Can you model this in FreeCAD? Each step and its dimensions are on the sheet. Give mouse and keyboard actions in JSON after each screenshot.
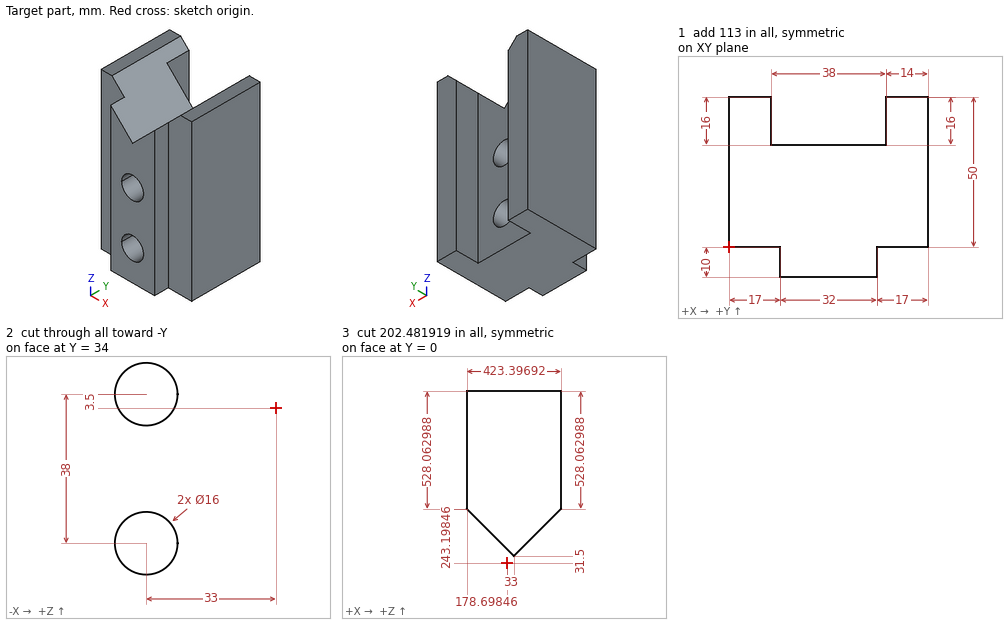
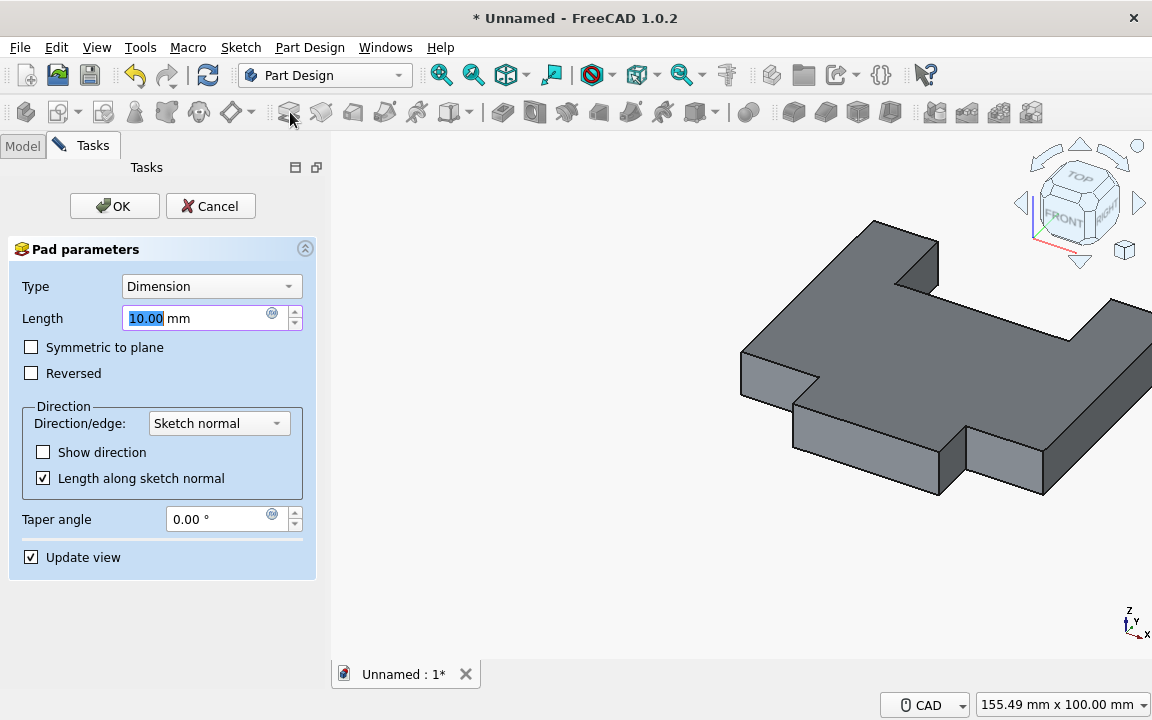
{"action": "type", "text": "113"}
{"action": "key", "text": "Tab"}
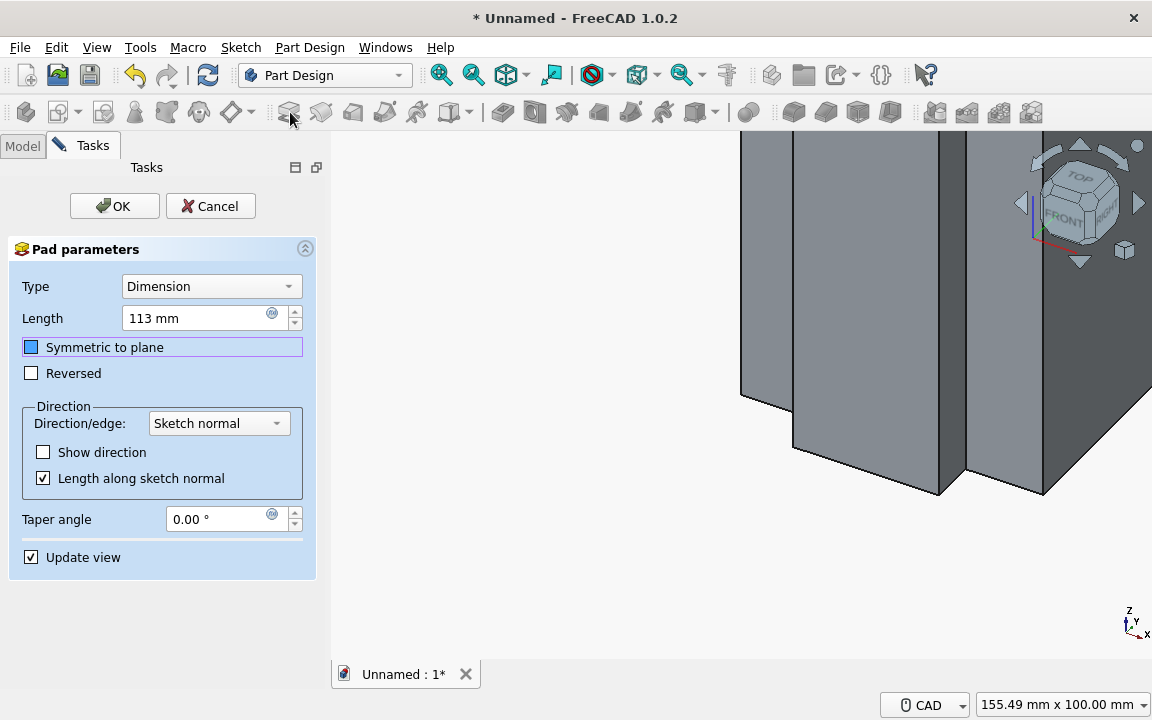
{"action": "left_click", "coordinate": [30, 347]}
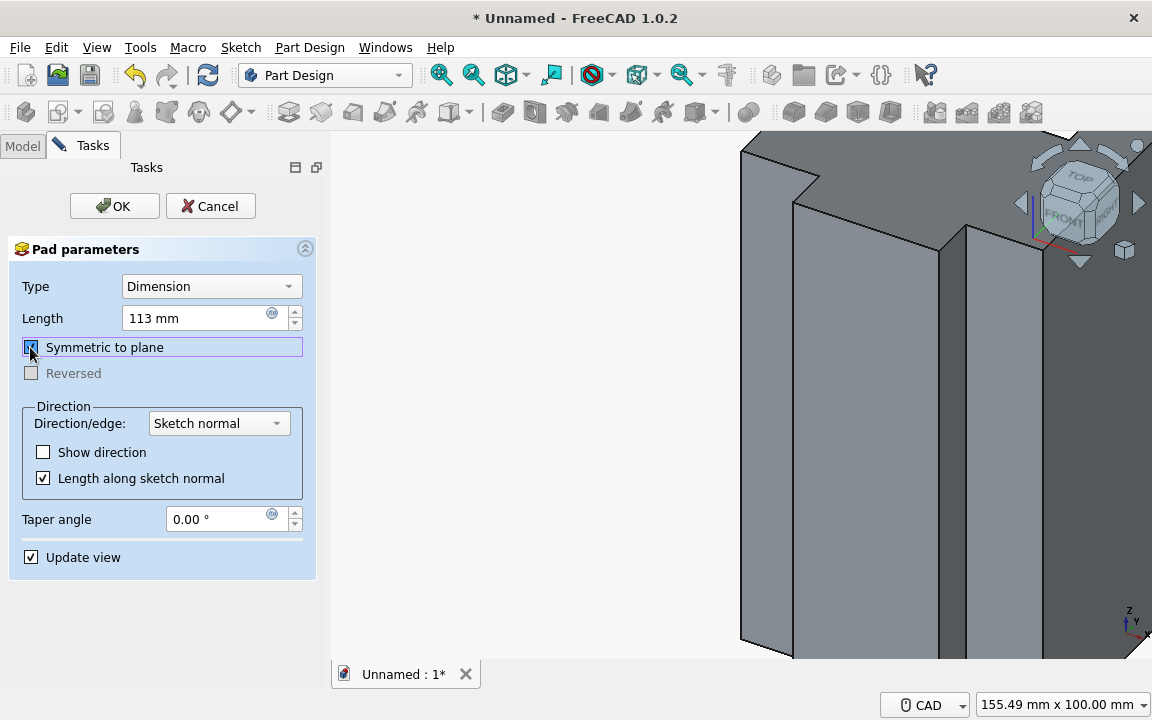
{"action": "left_click", "coordinate": [115, 206]}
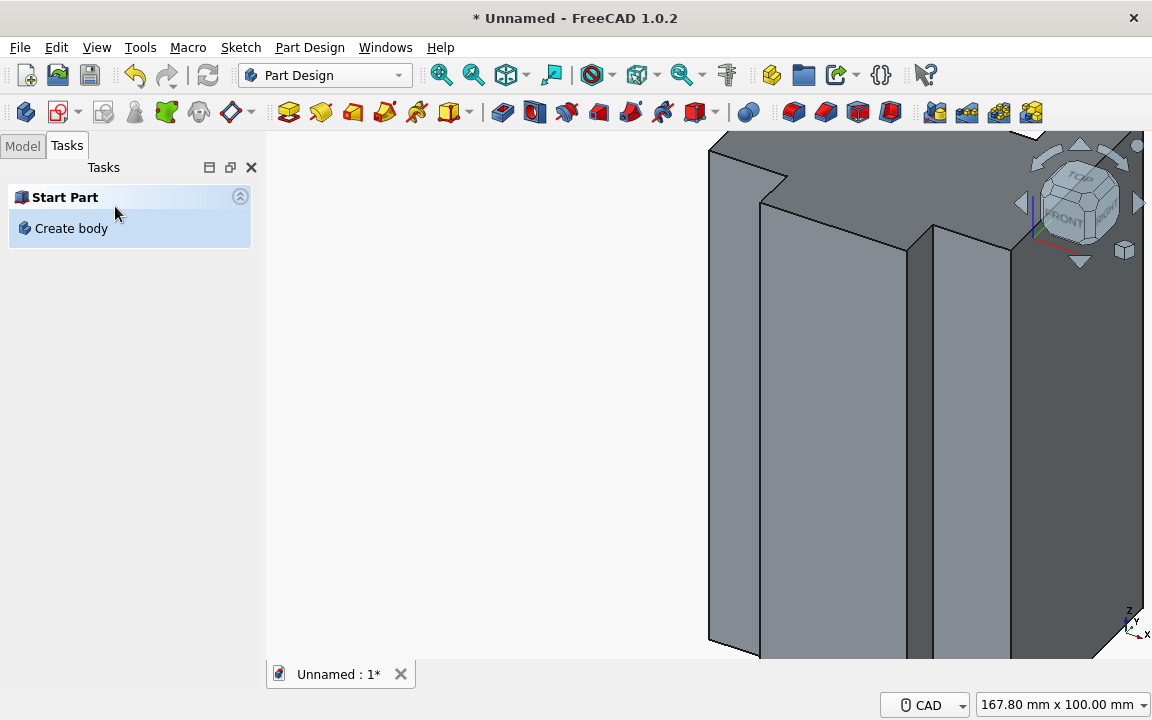
{"action": "left_click", "coordinate": [442, 76]}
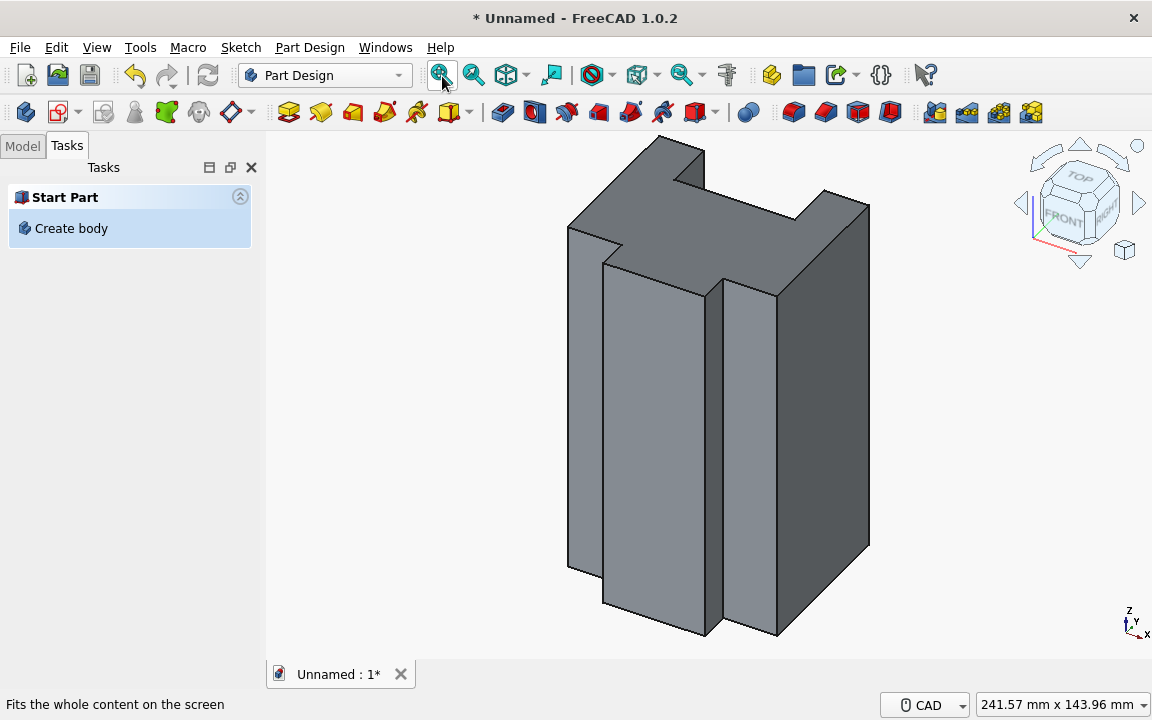
{"action": "key", "text": "4"}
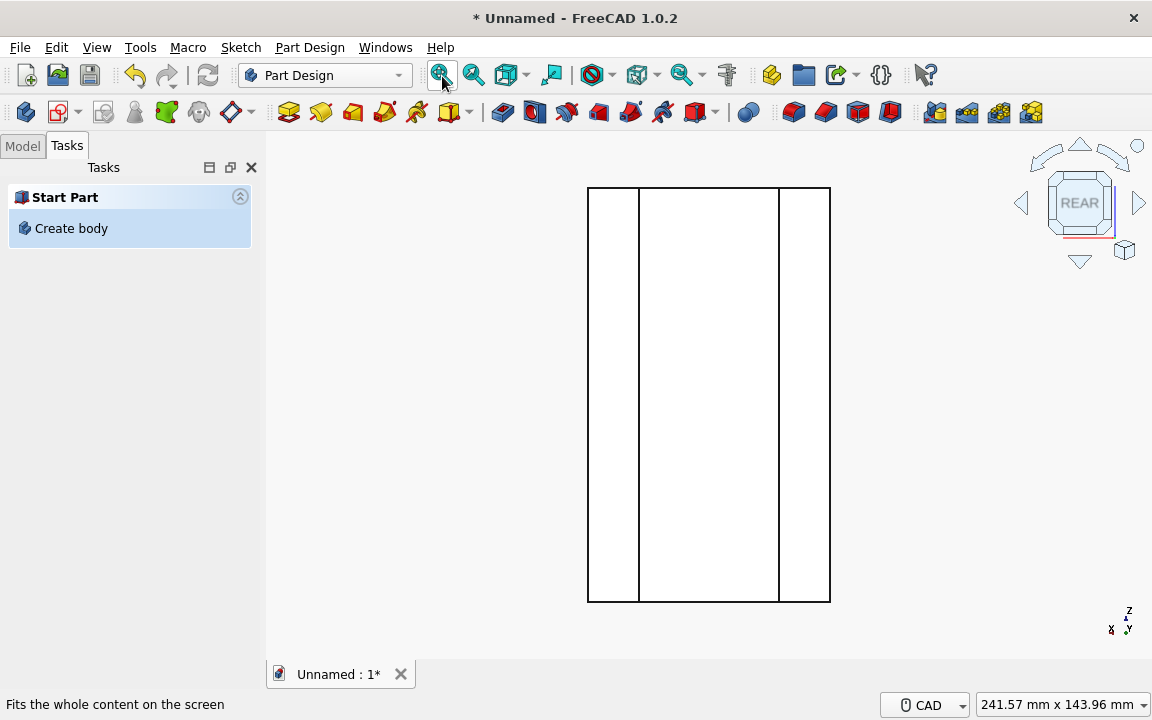
{"action": "left_click", "coordinate": [709, 276]}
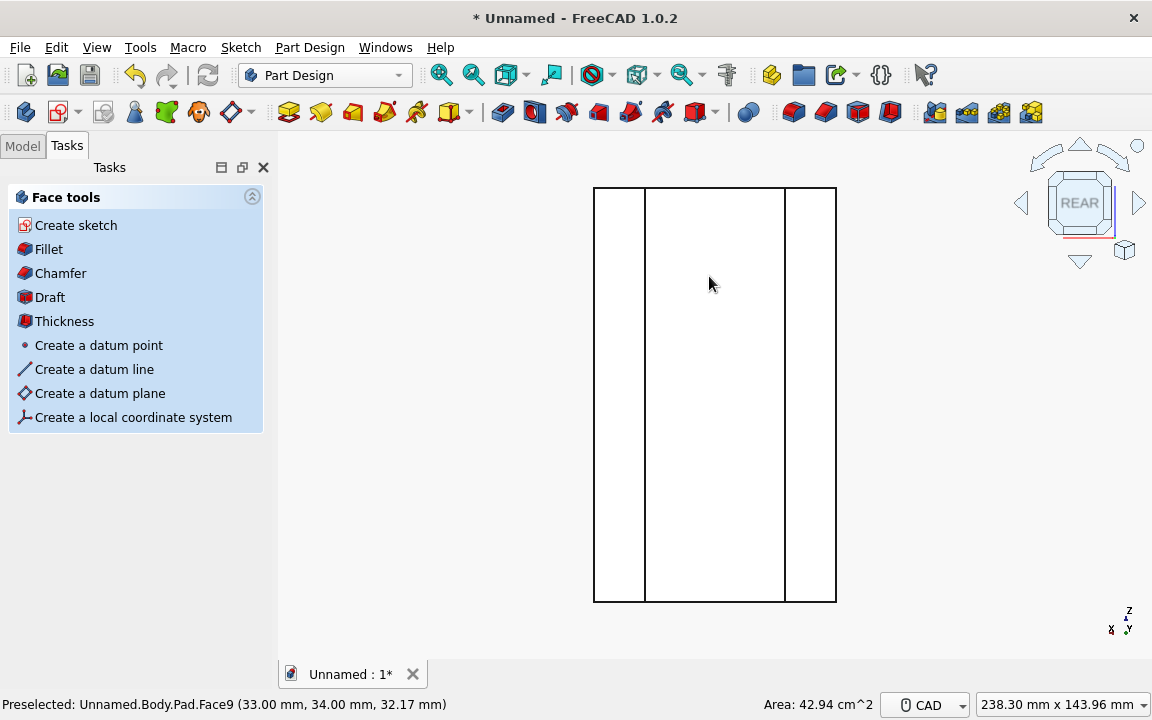
{"action": "left_click", "coordinate": [58, 112]}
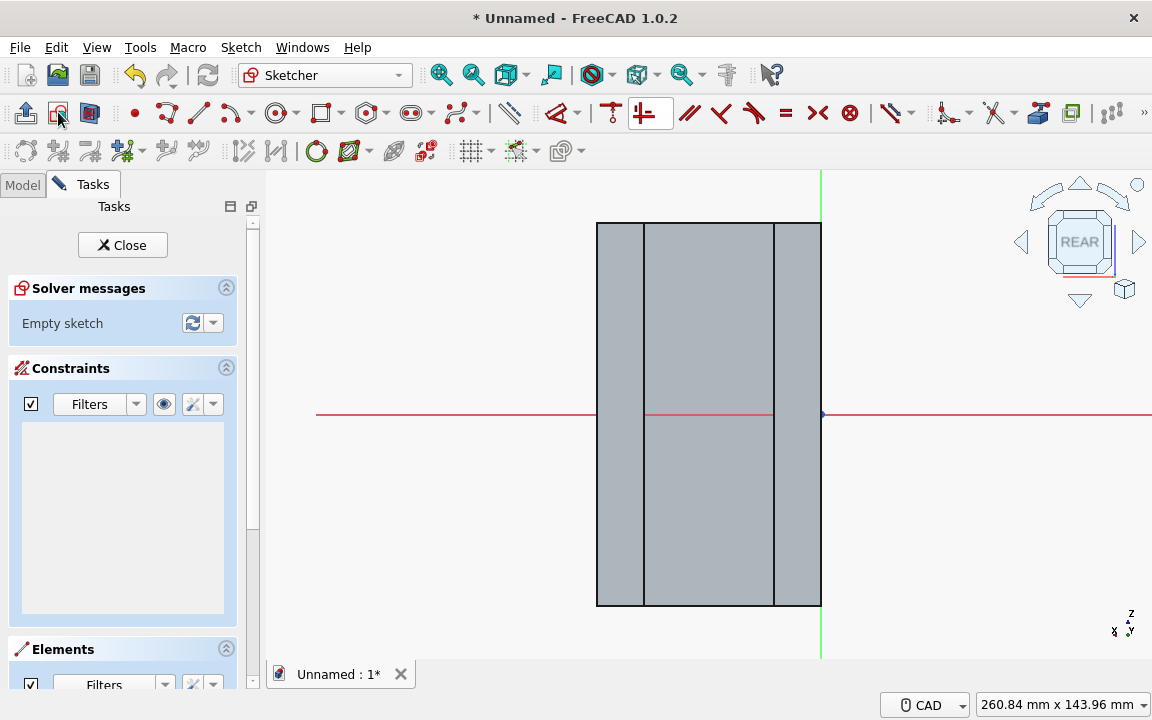
{"action": "scroll", "coordinate": [886, 531], "scroll_direction": "up", "scroll_amount": 3}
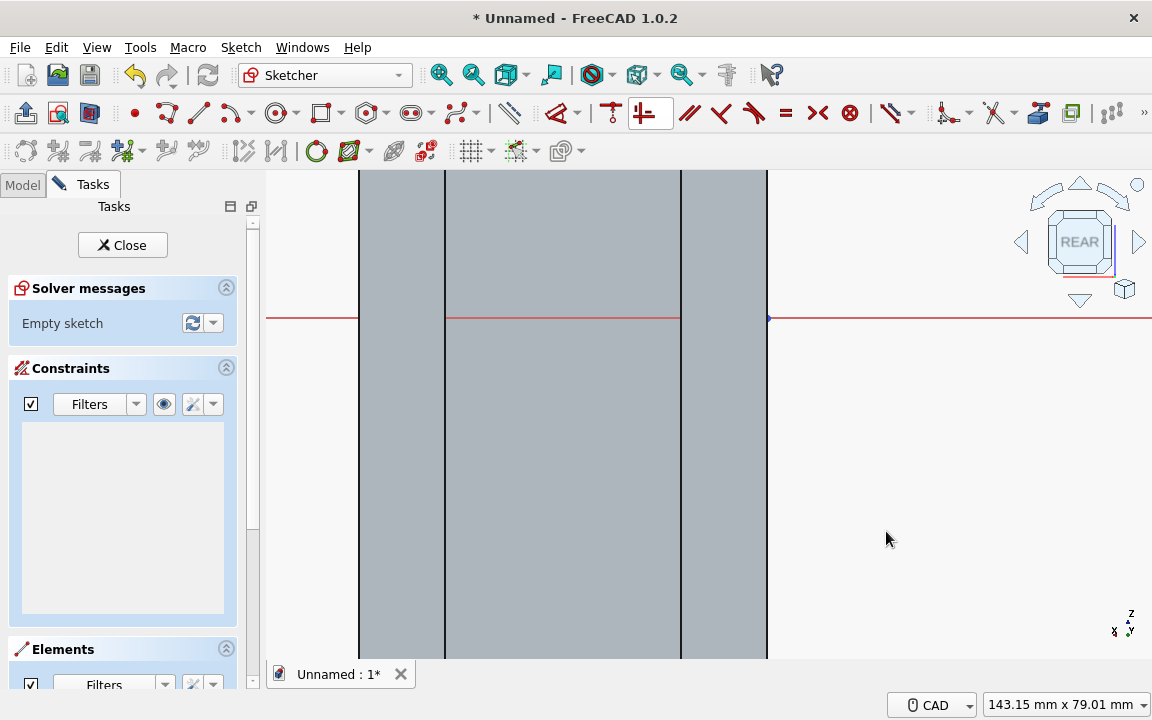
{"action": "left_click", "coordinate": [276, 114]}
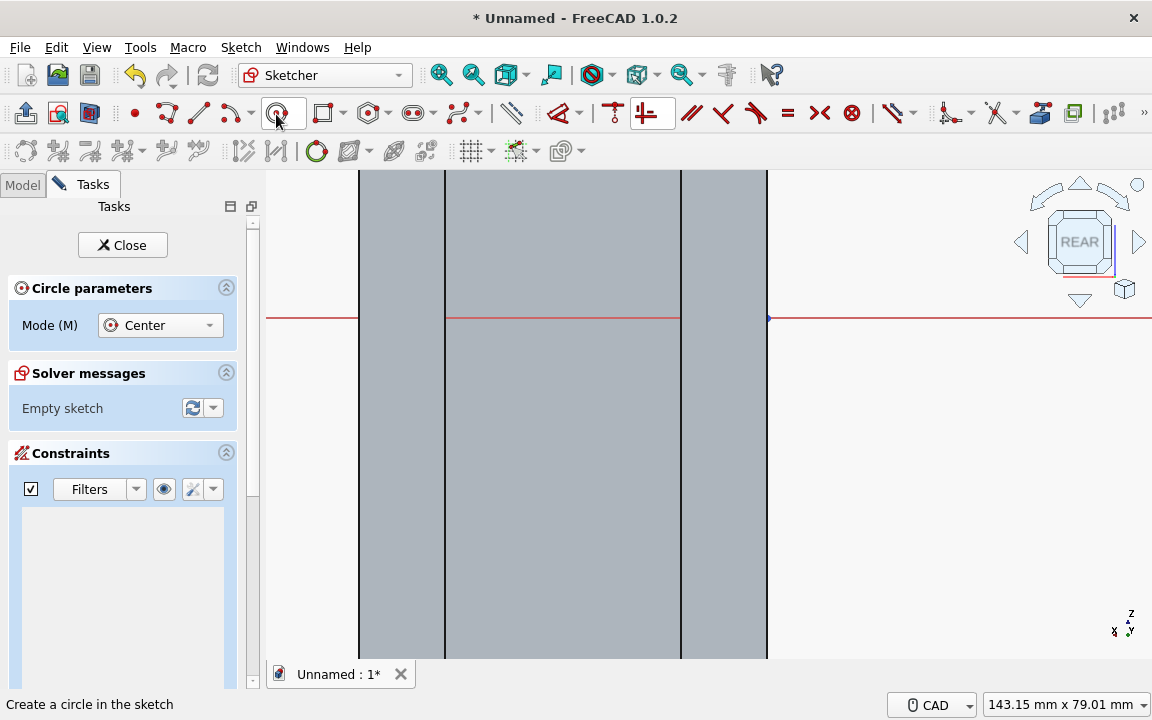
{"action": "left_click", "coordinate": [563, 532]}
{"action": "left_click", "coordinate": [598, 497]}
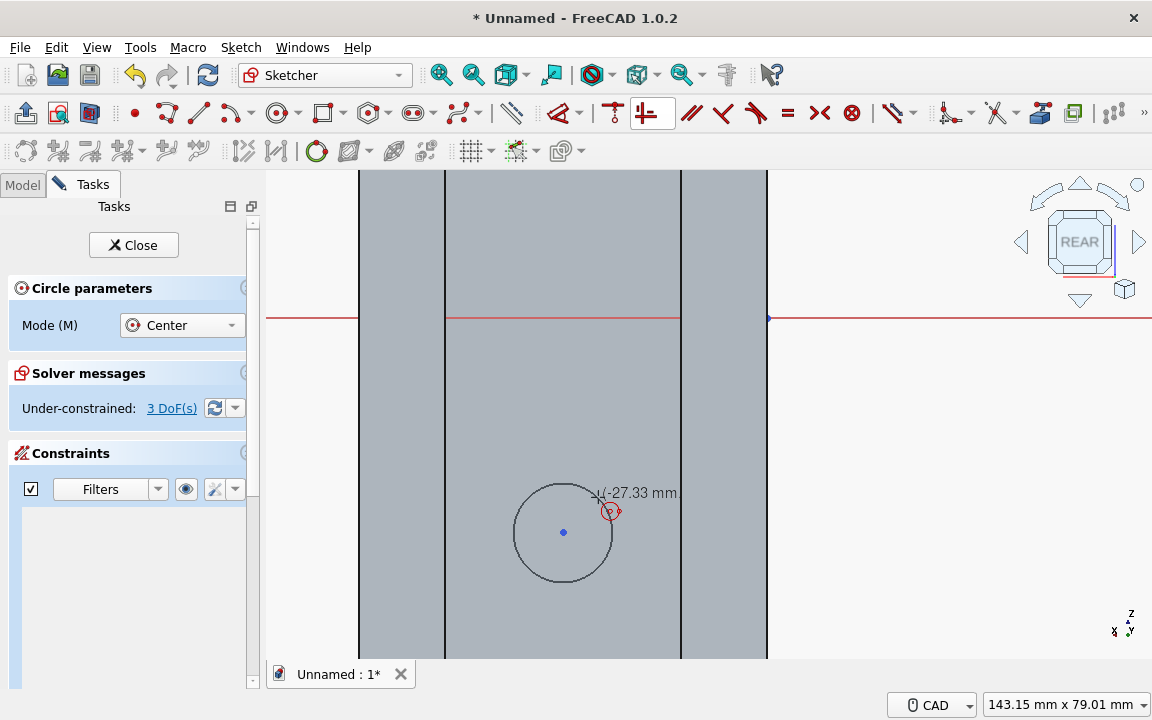
{"action": "left_click", "coordinate": [563, 296]}
{"action": "left_click", "coordinate": [598, 261]}
{"action": "key", "text": "Escape"}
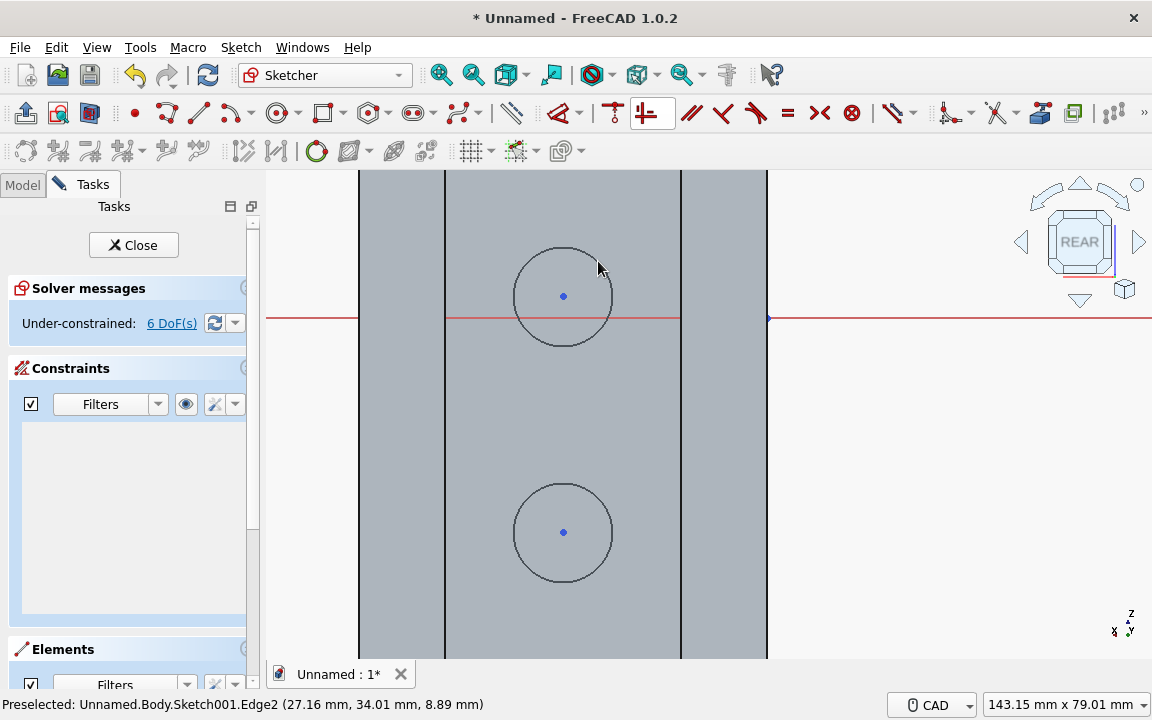
{"action": "left_click", "coordinate": [598, 498]}